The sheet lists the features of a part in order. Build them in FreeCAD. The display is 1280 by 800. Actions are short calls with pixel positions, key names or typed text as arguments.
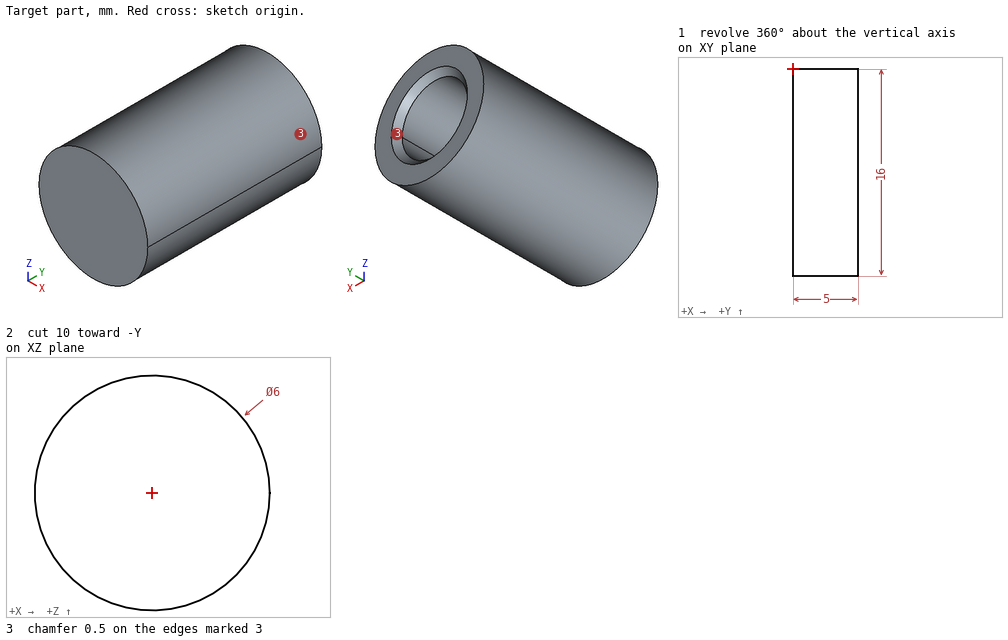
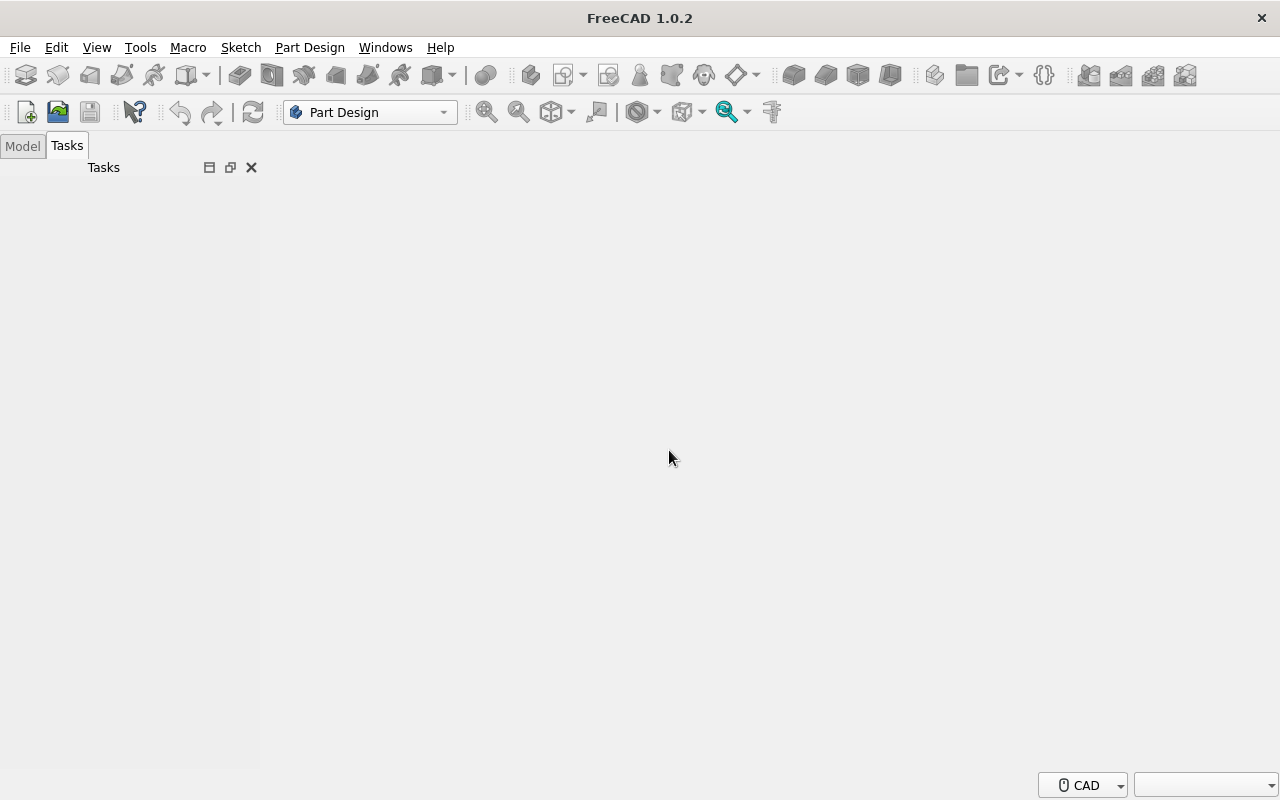
key(ctrl+n)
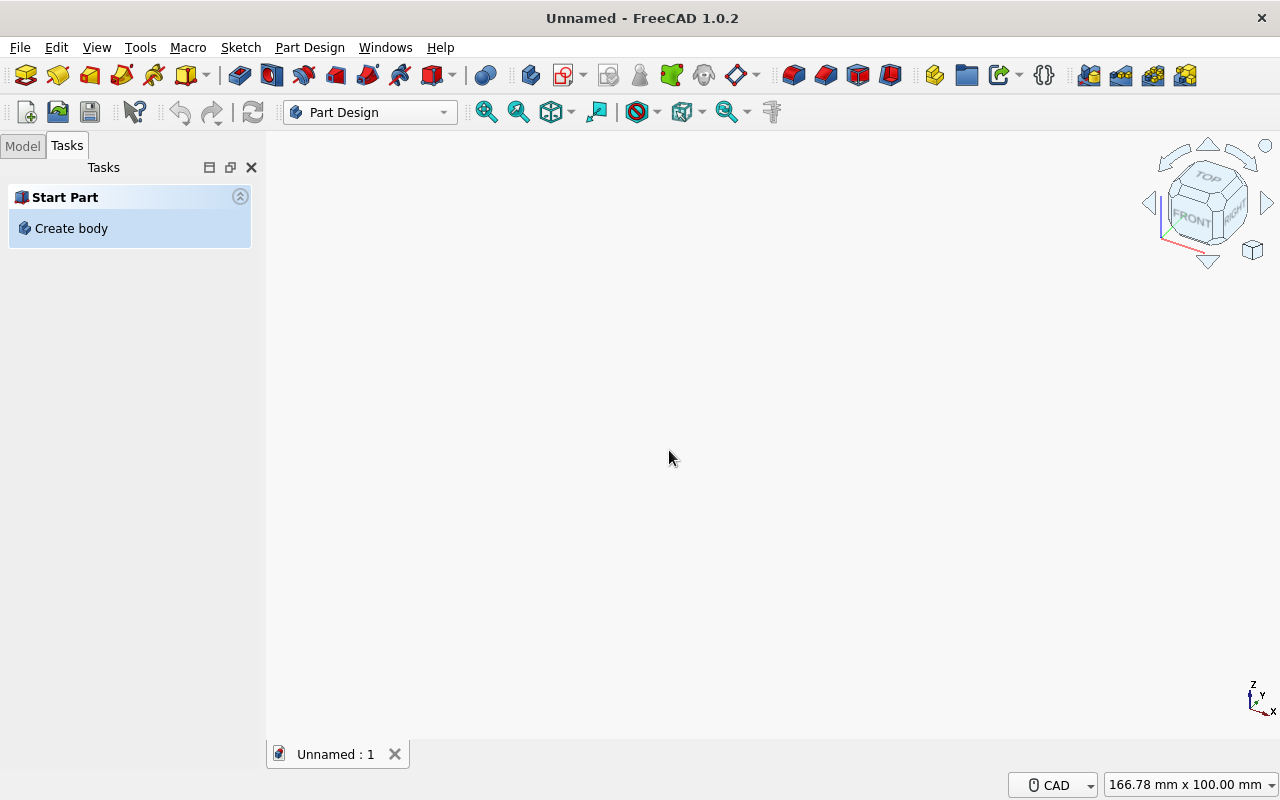
click(564, 76)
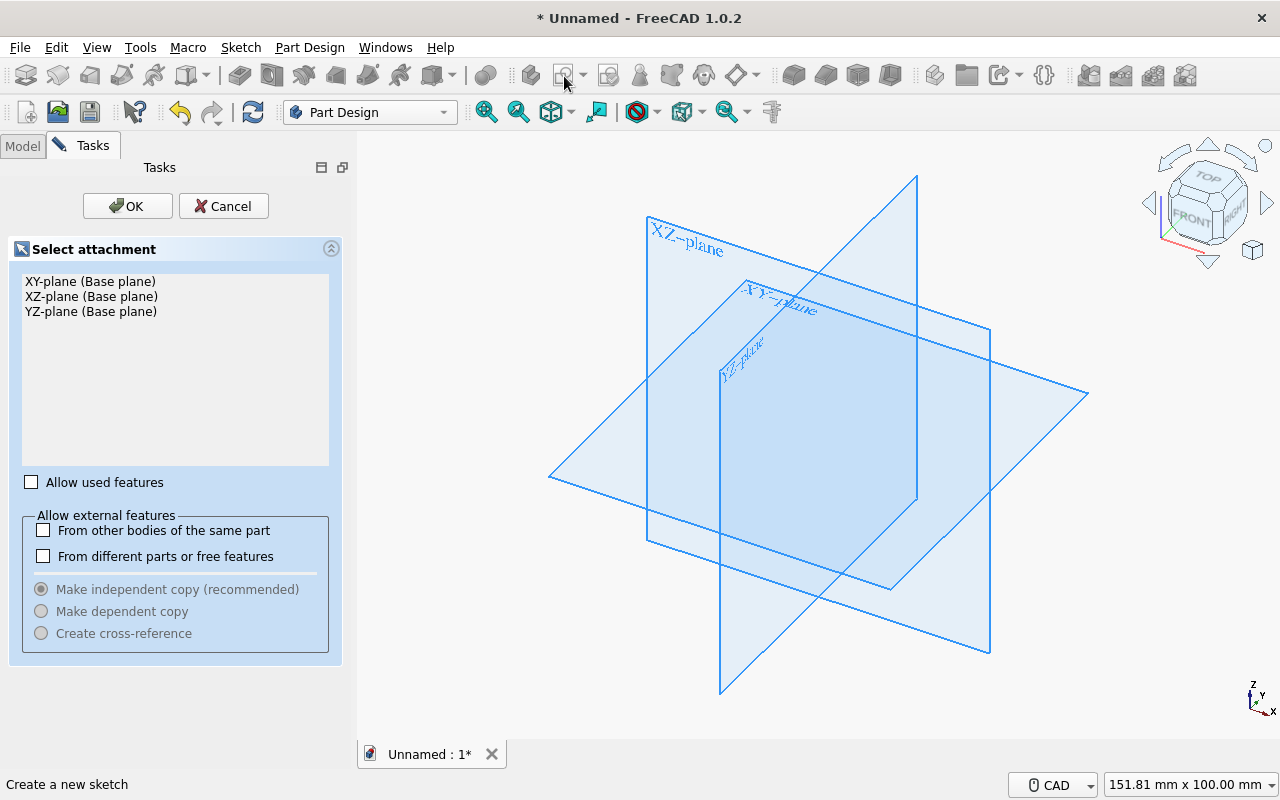
click(82, 282)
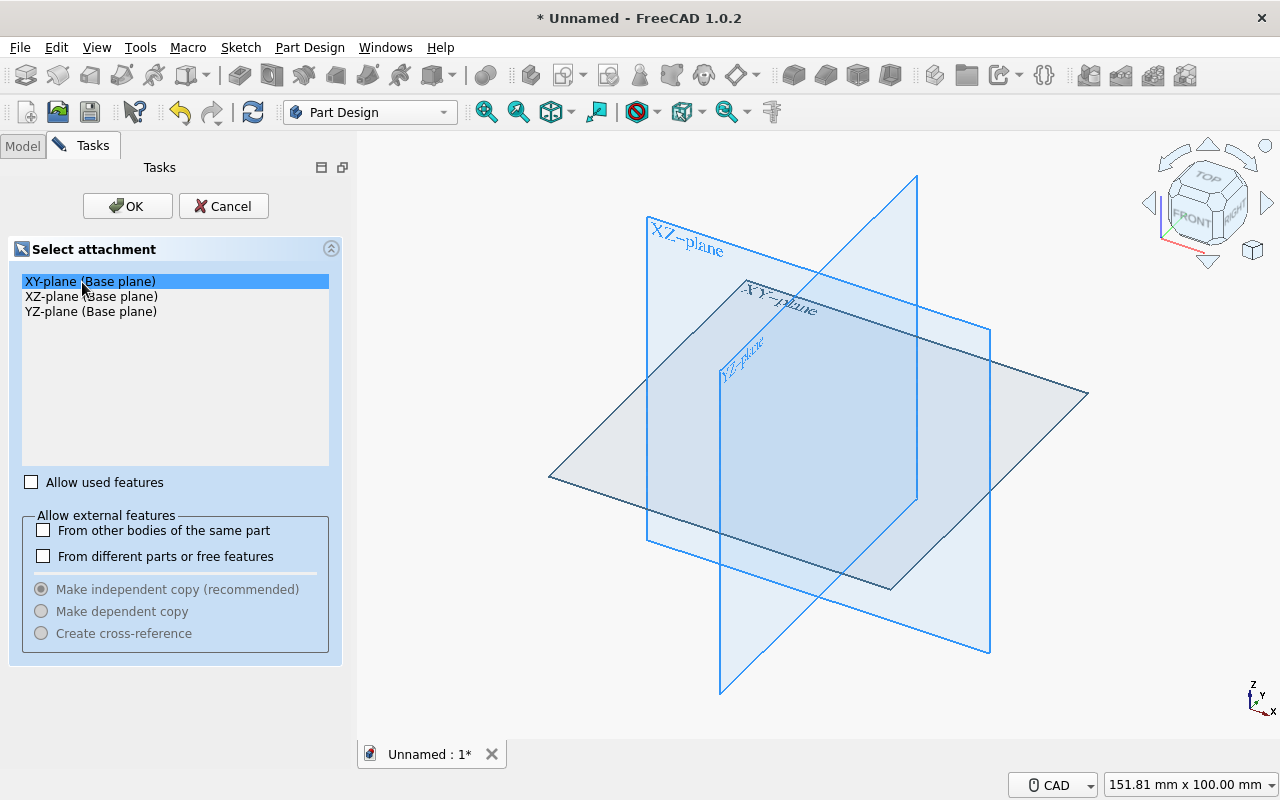
click(128, 206)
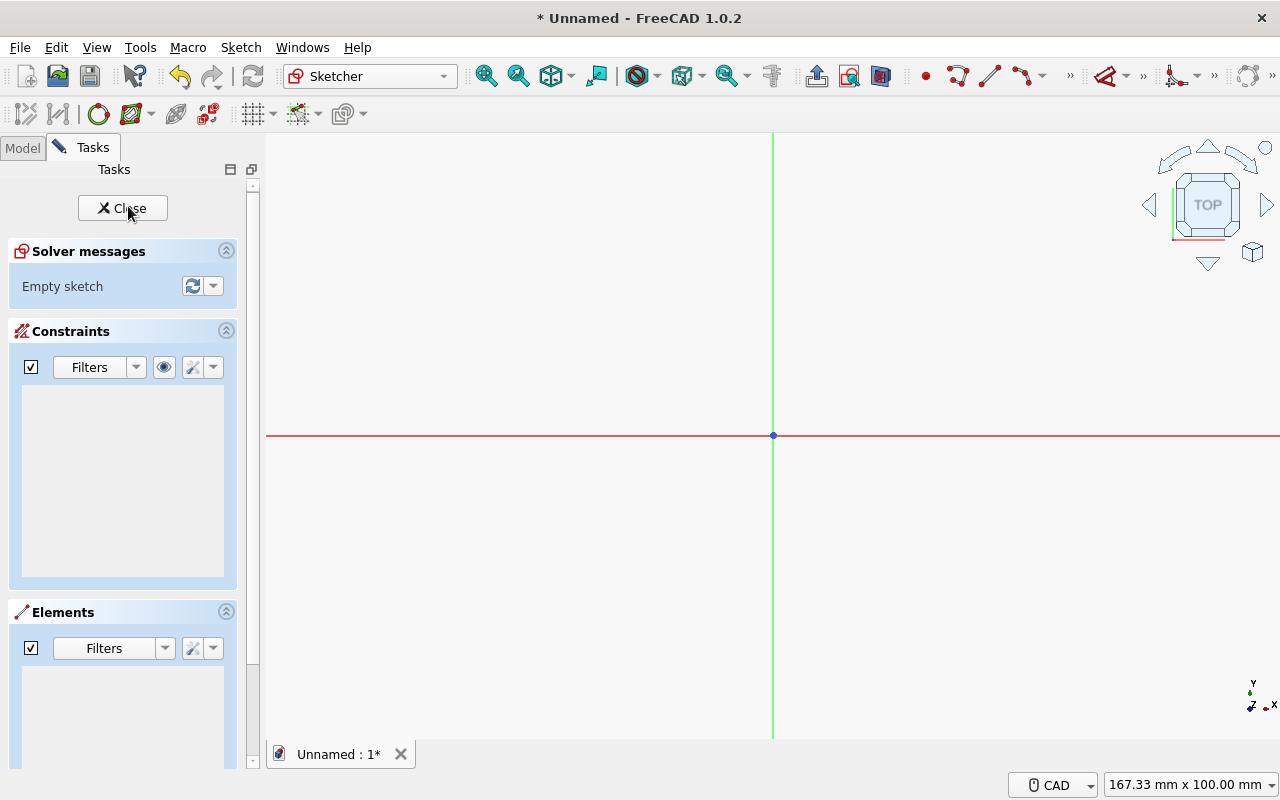
scroll(816, 500, up, 7)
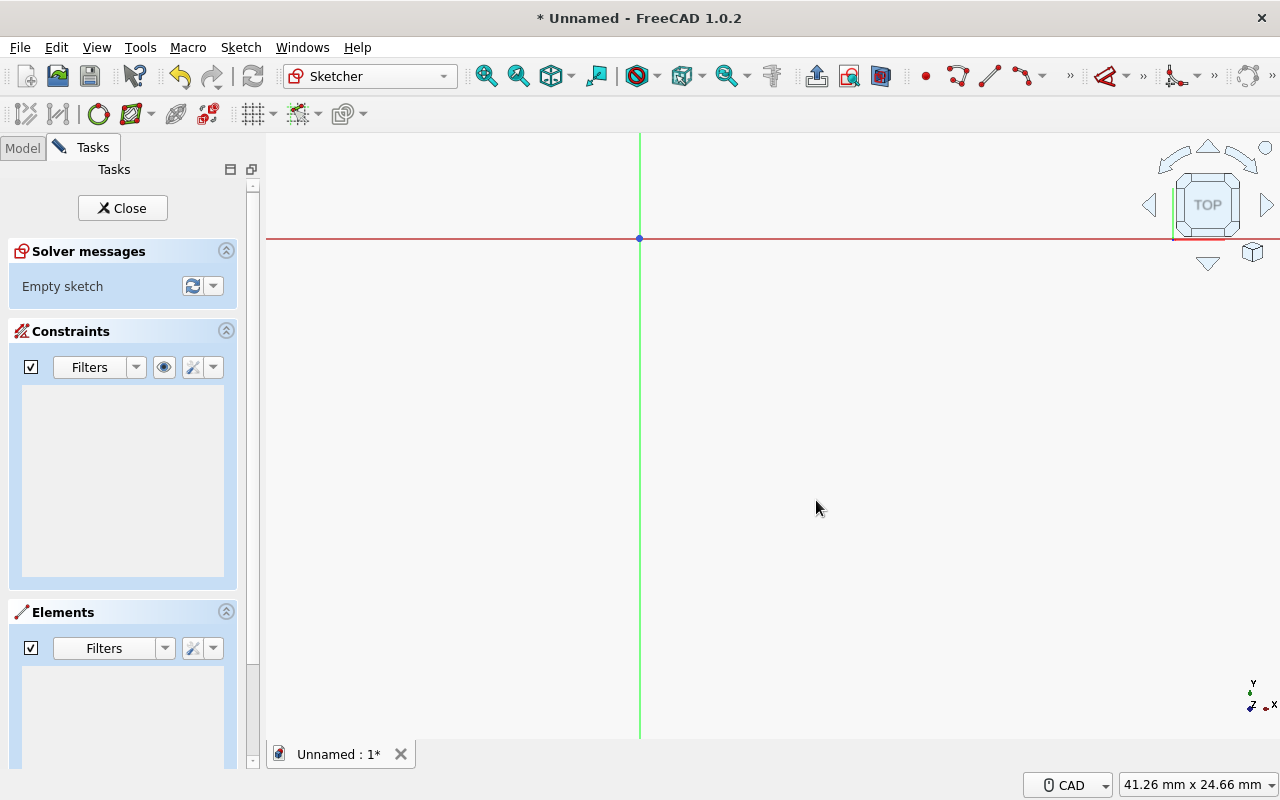
key(g)
key(r)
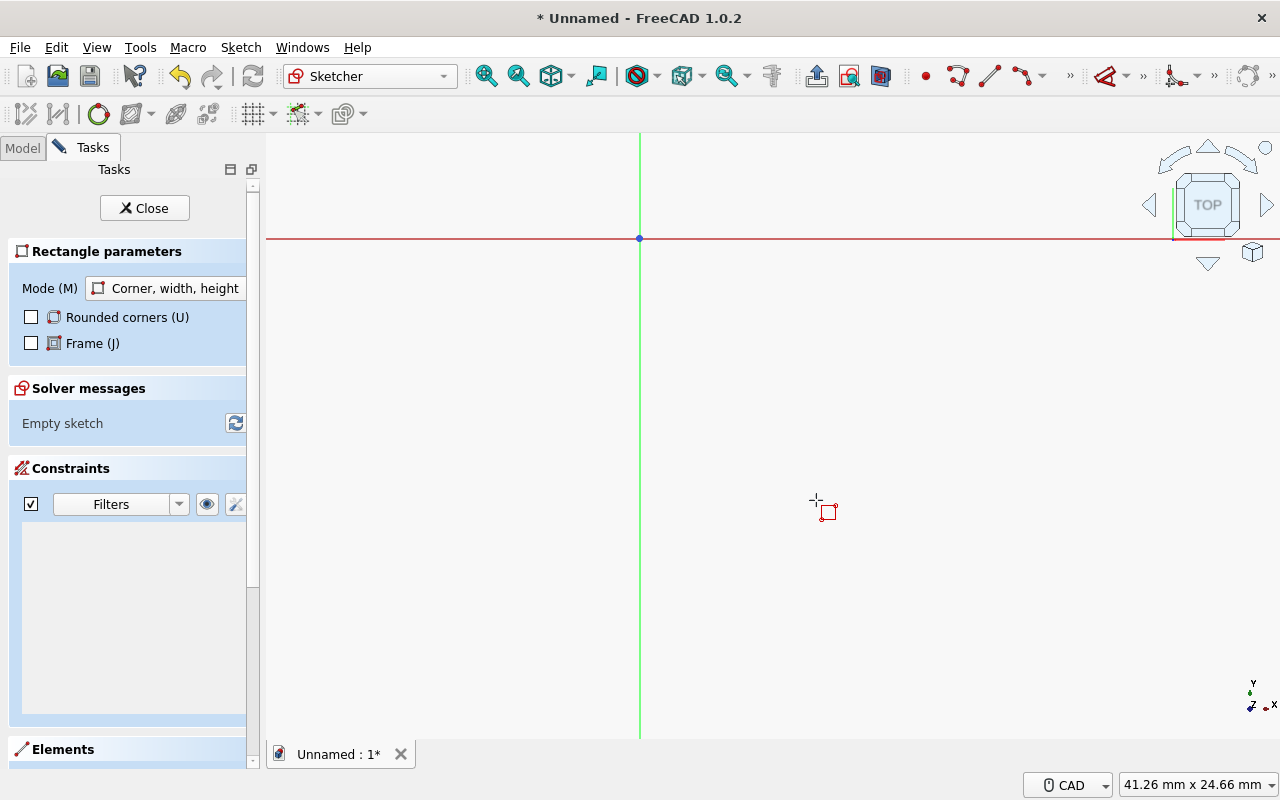
click(640, 239)
move(763, 632)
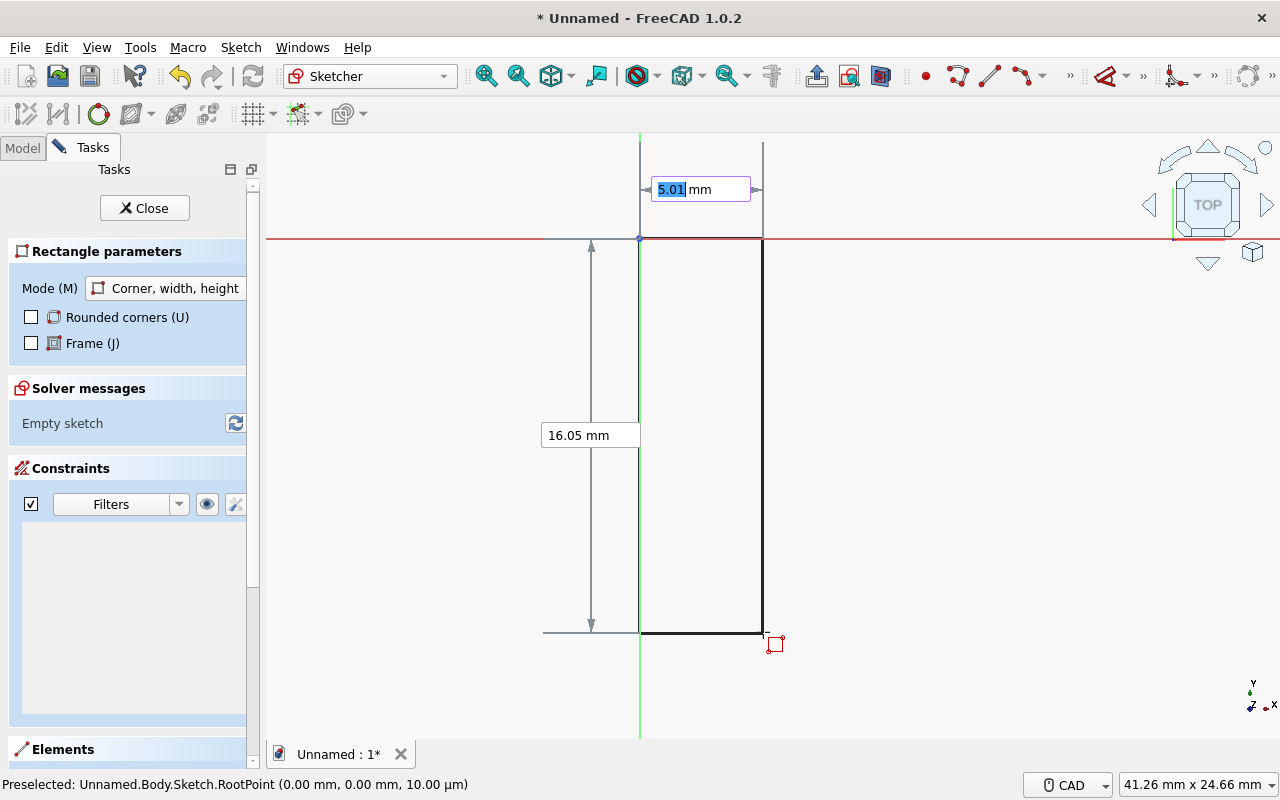
text(5)
key(Tab)
text(16)
key(Return)
key(Escape)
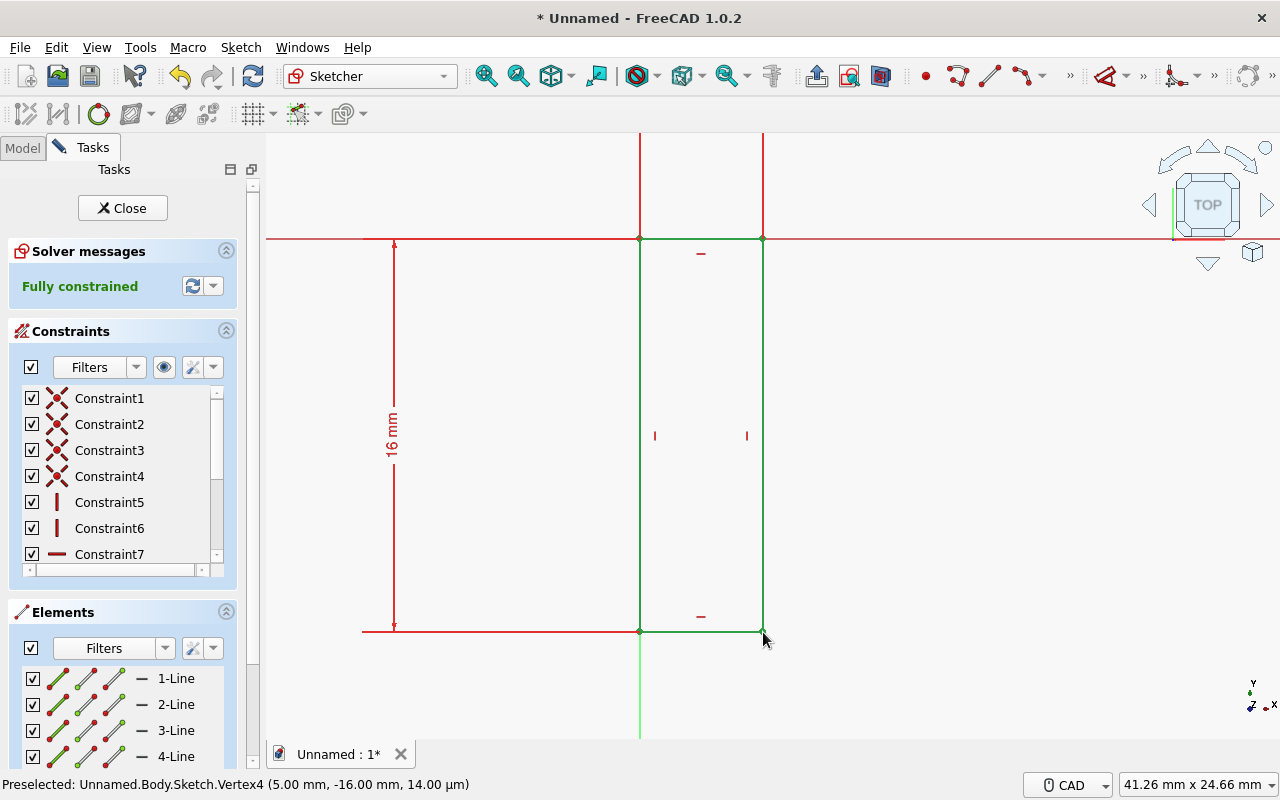
click(123, 208)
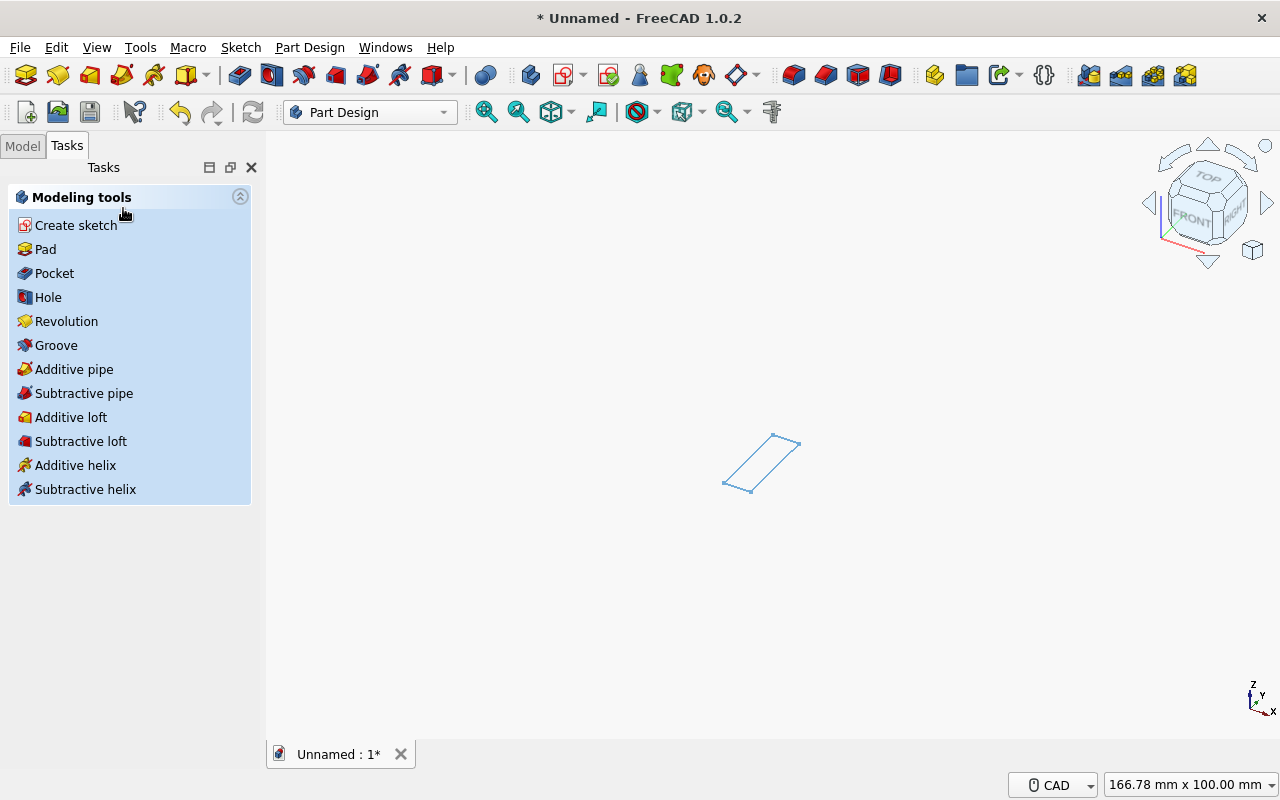
click(58, 76)